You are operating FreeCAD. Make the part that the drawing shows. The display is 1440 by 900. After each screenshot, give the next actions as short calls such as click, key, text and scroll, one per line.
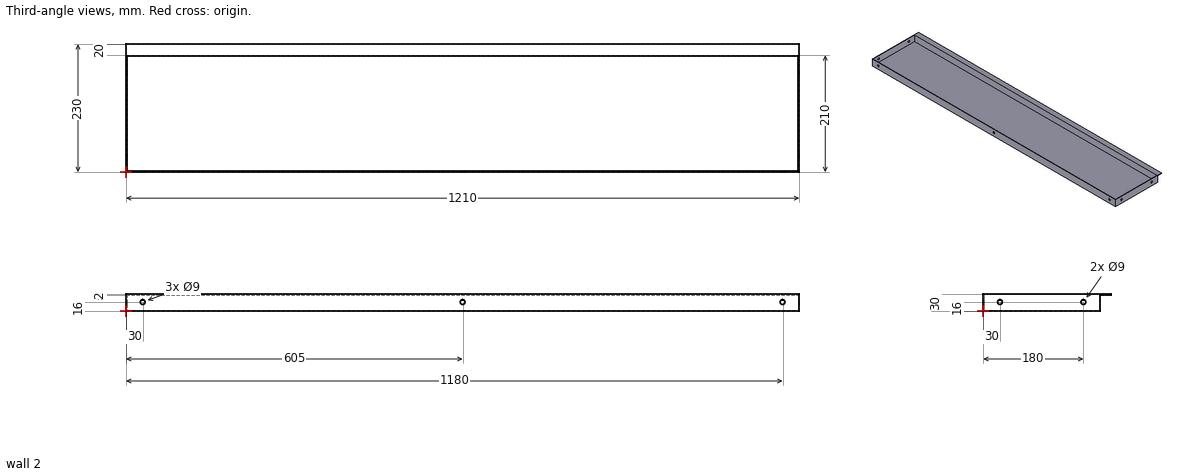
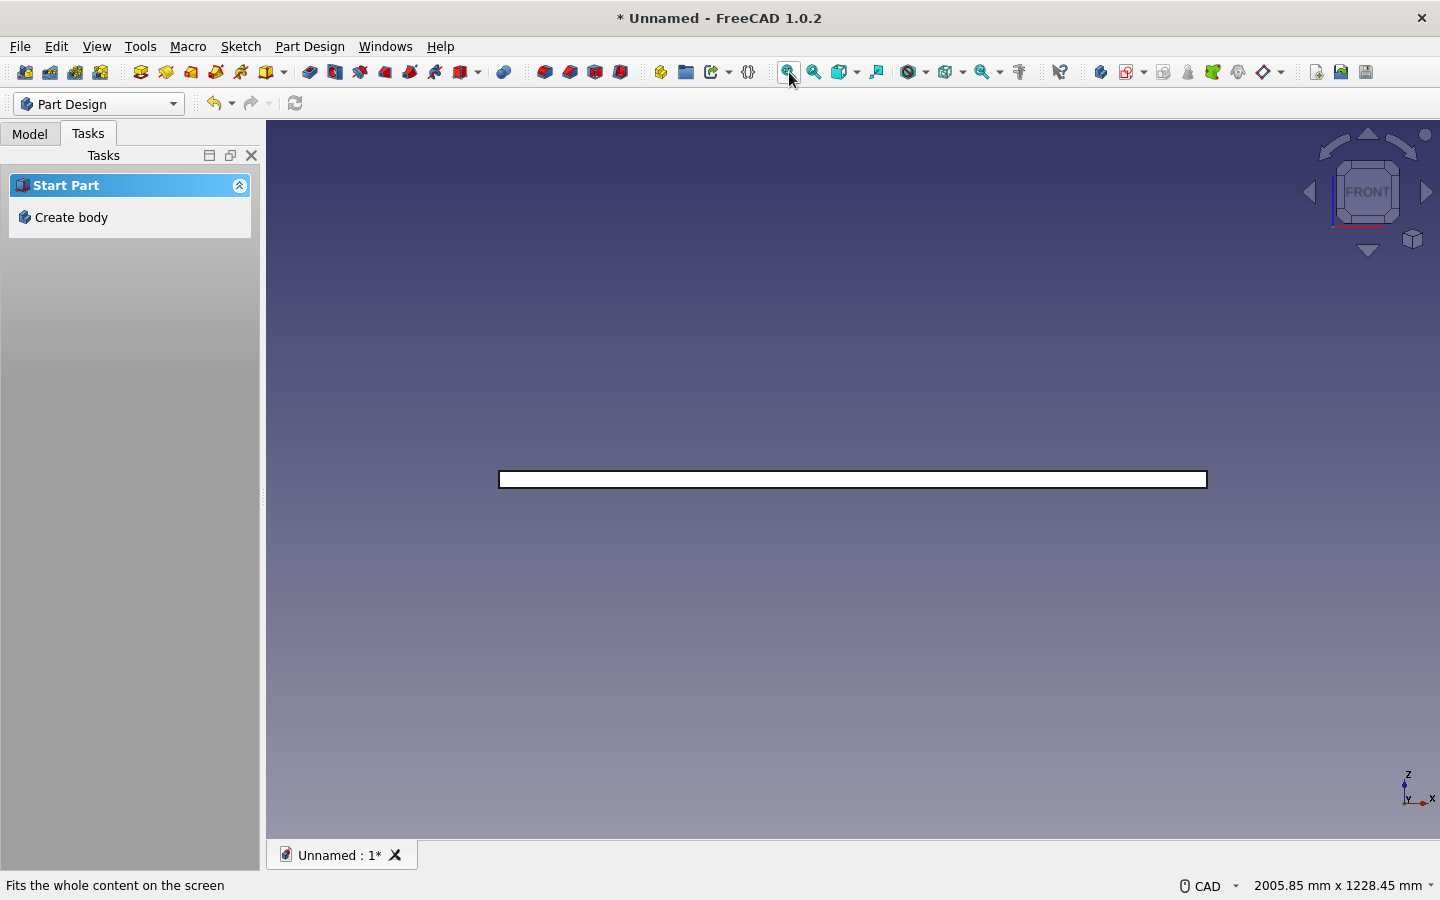
click(30, 134)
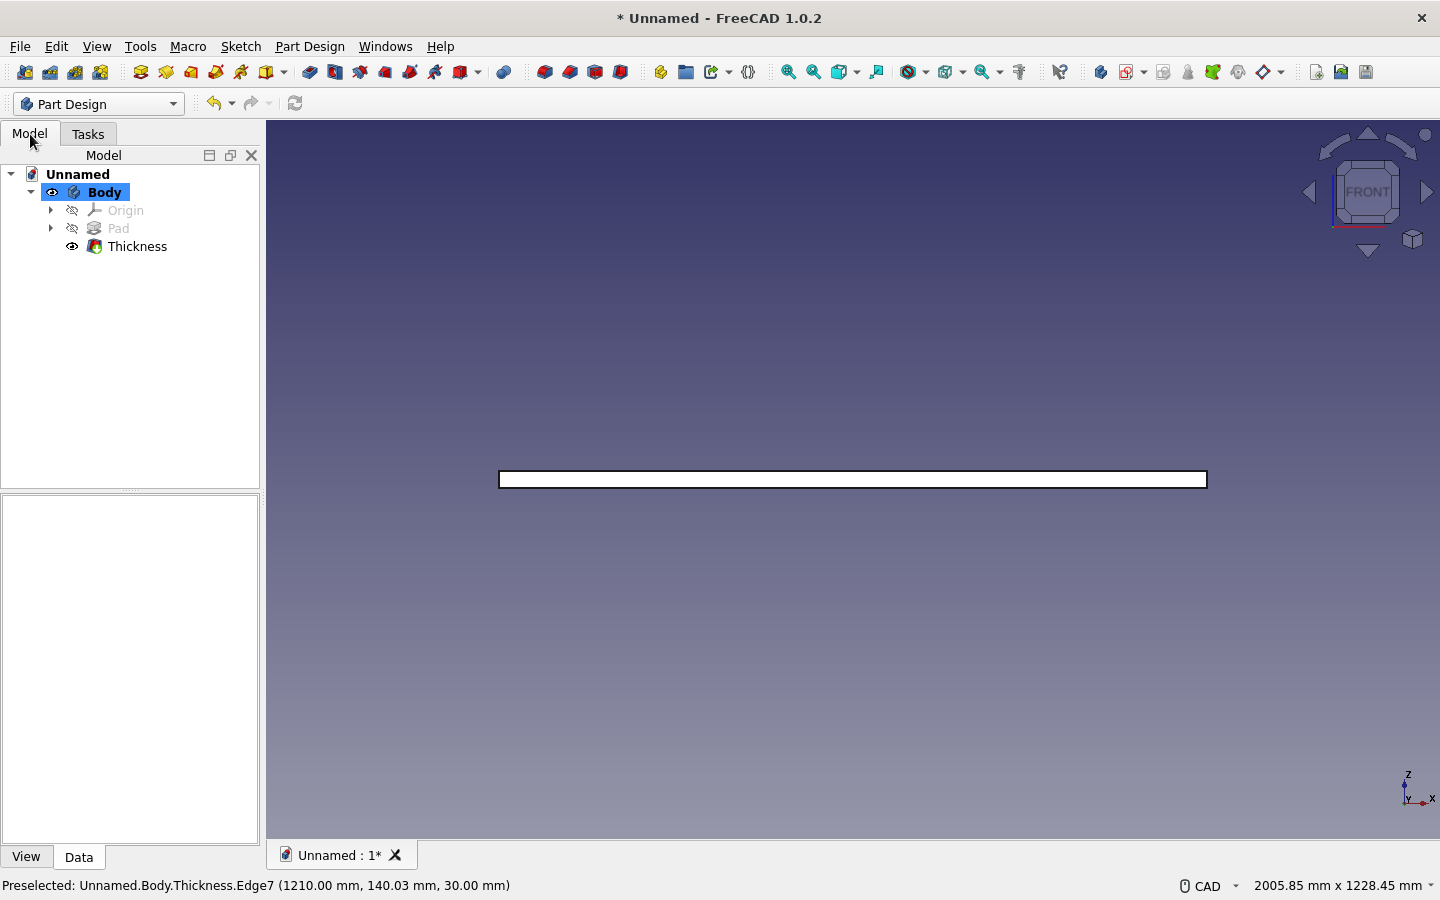
click(51, 210)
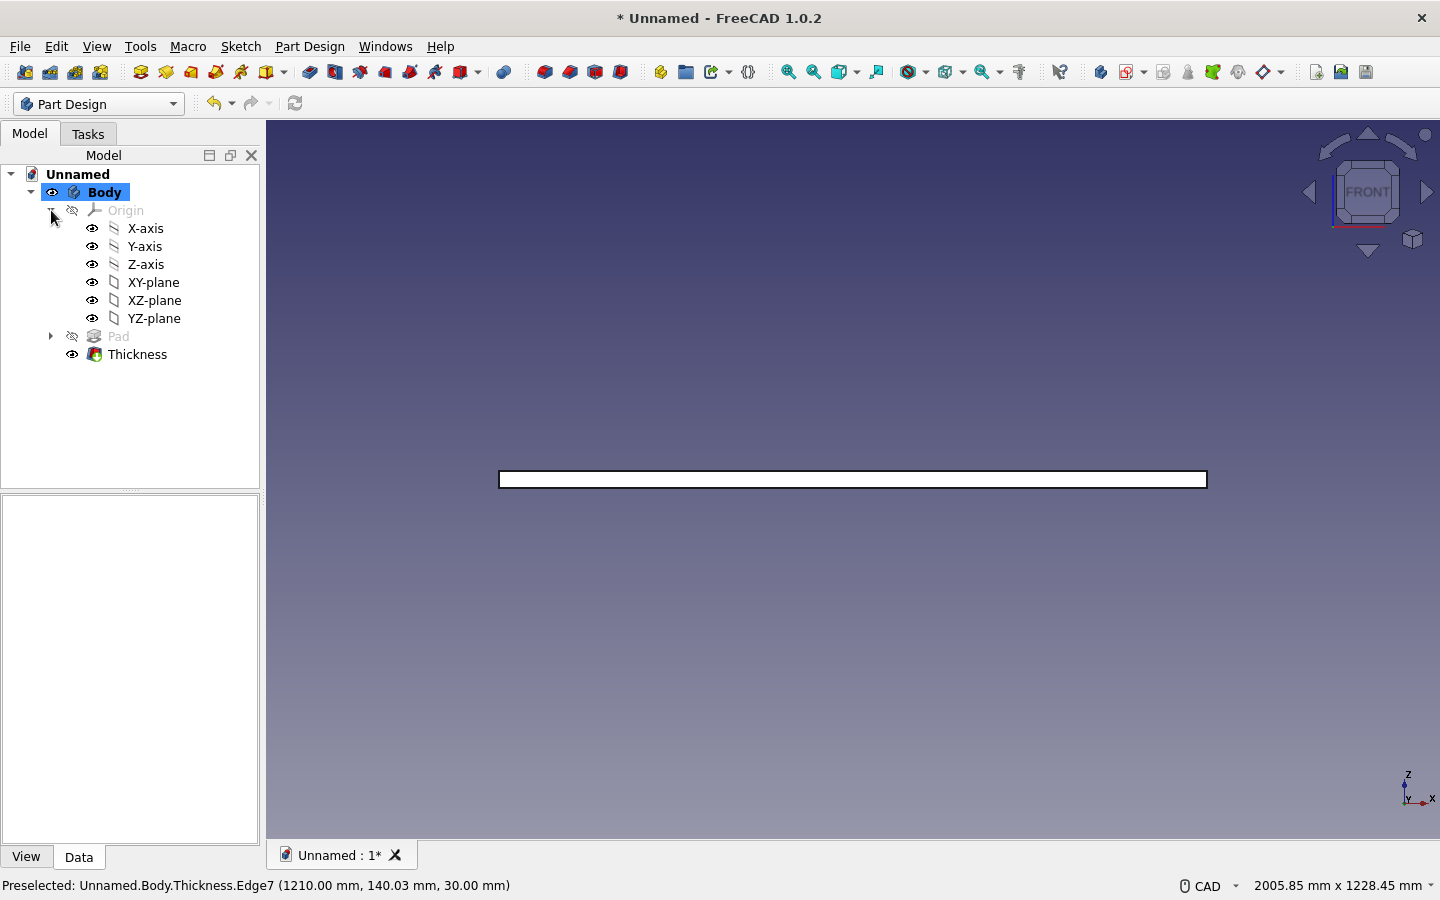
click(137, 282)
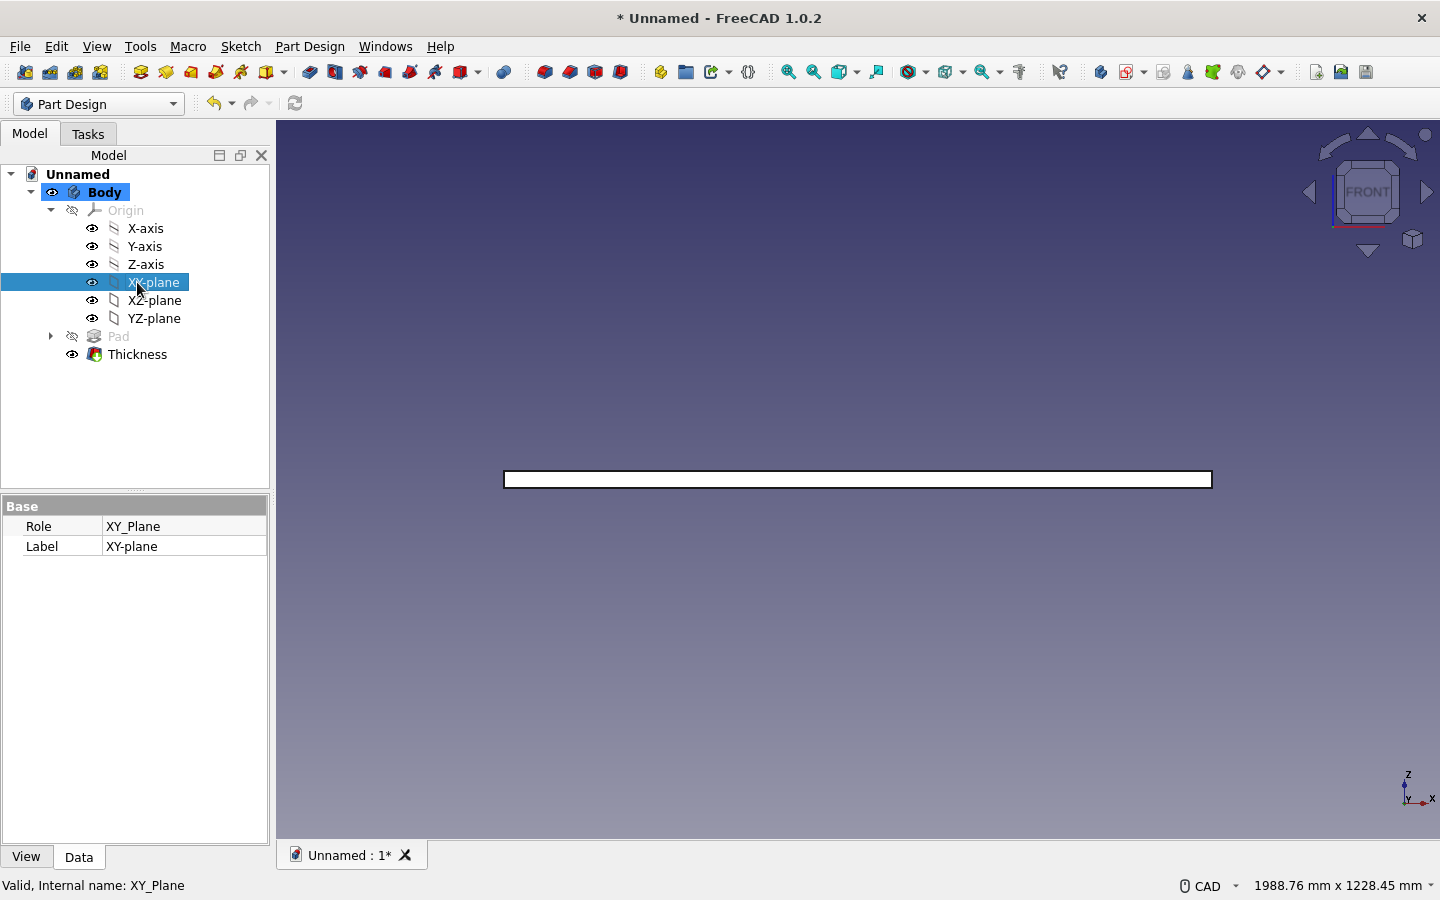
click(1262, 72)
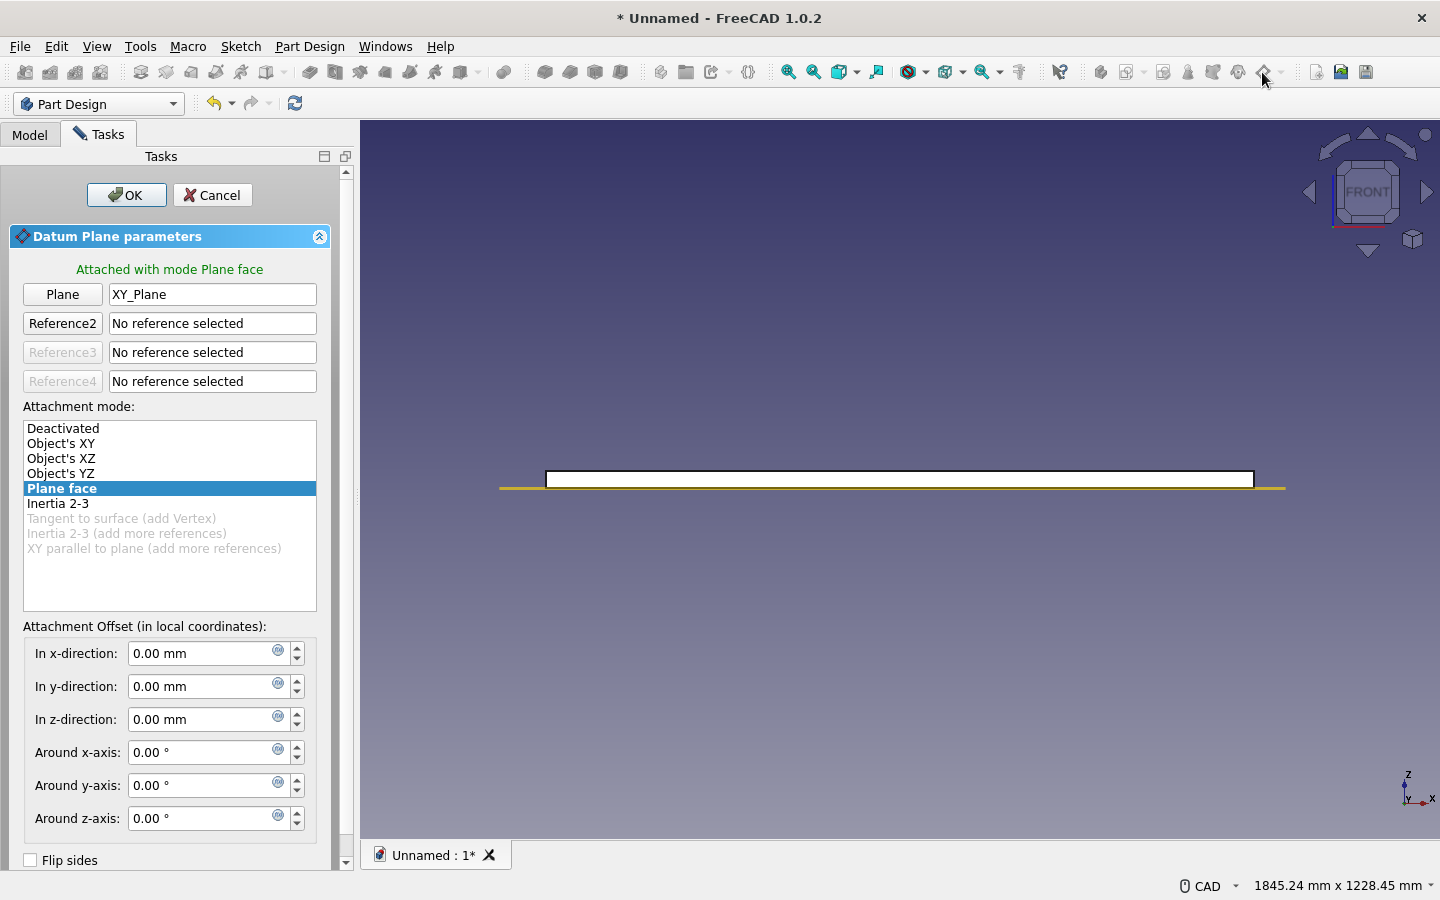
triple_click(210, 720)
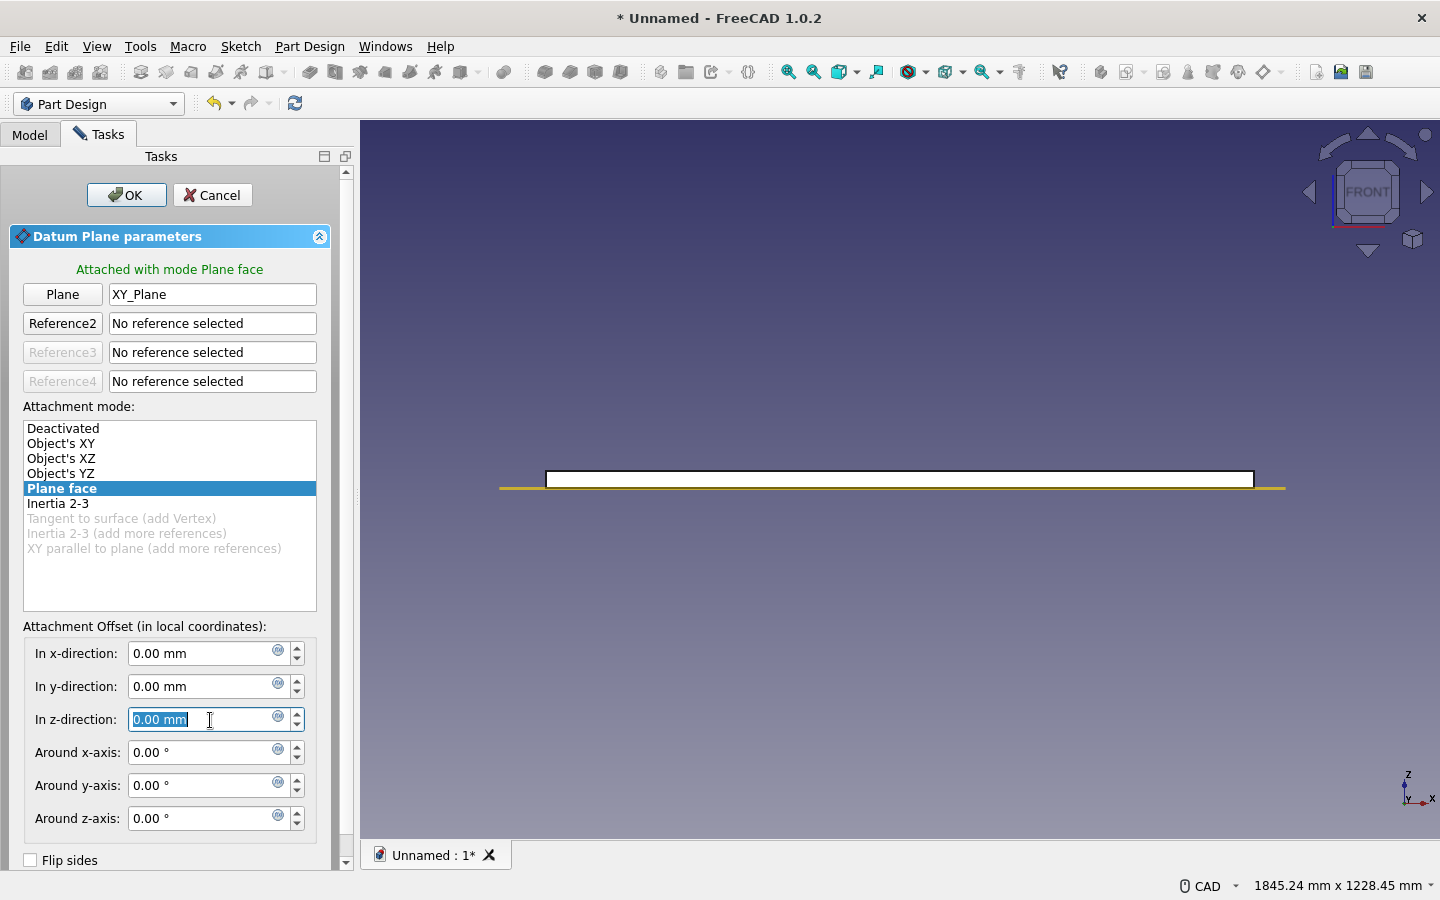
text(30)
key(Tab)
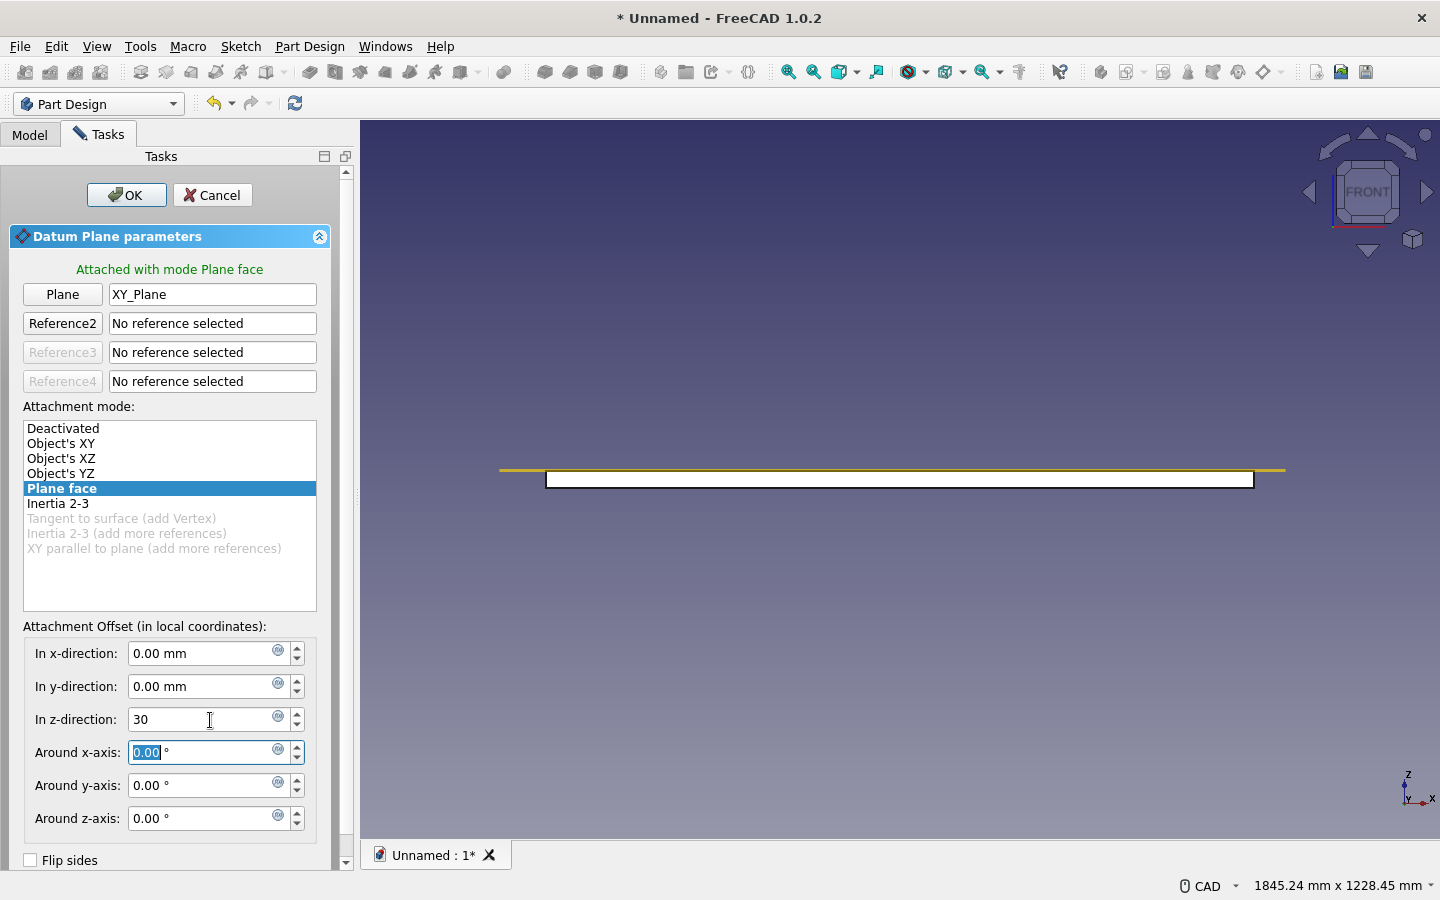
click(127, 195)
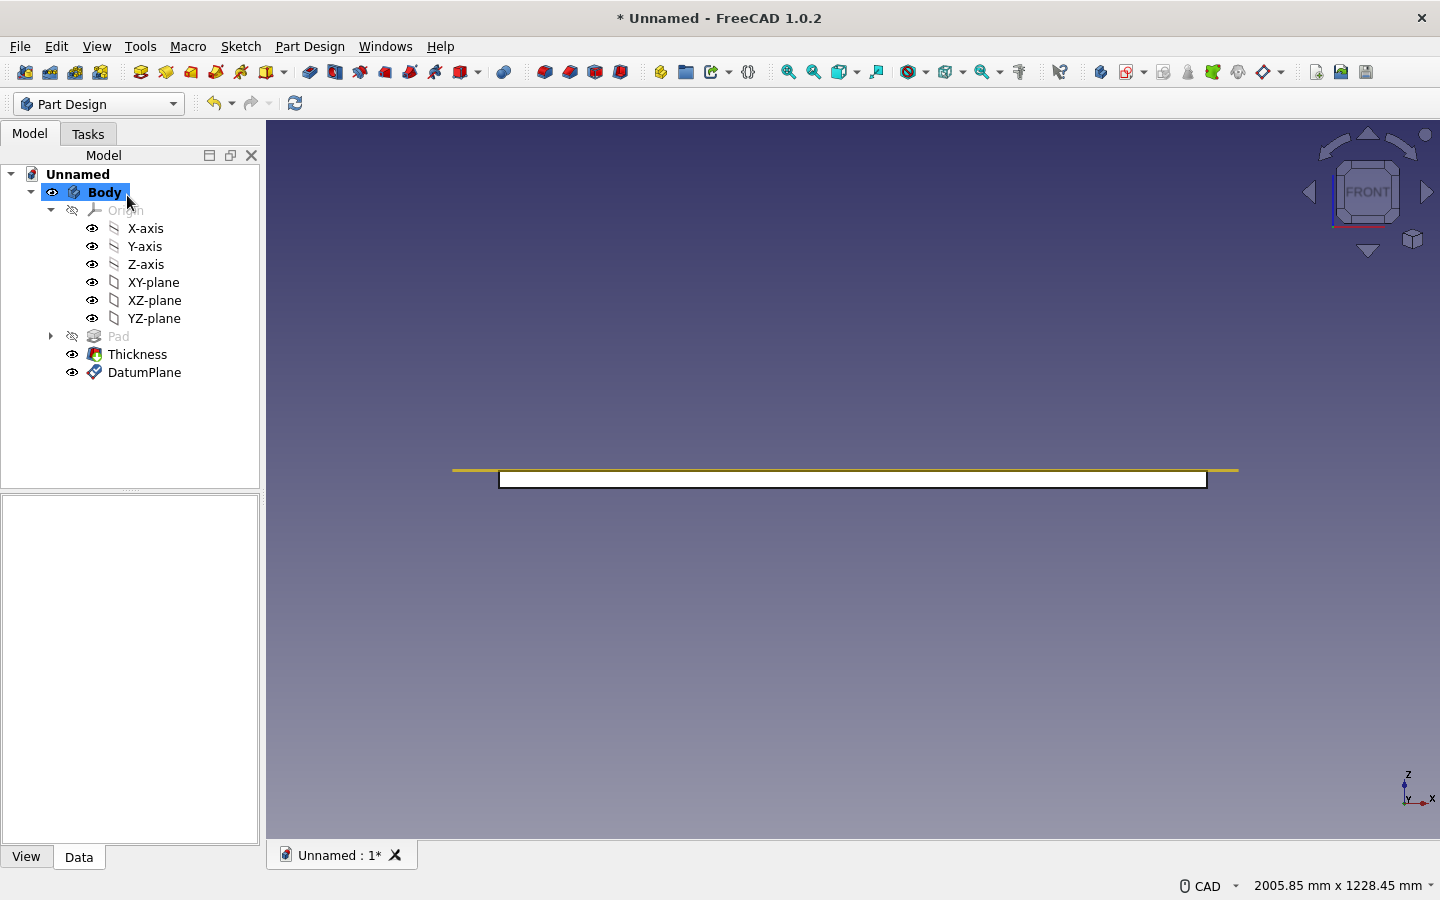
click(117, 372)